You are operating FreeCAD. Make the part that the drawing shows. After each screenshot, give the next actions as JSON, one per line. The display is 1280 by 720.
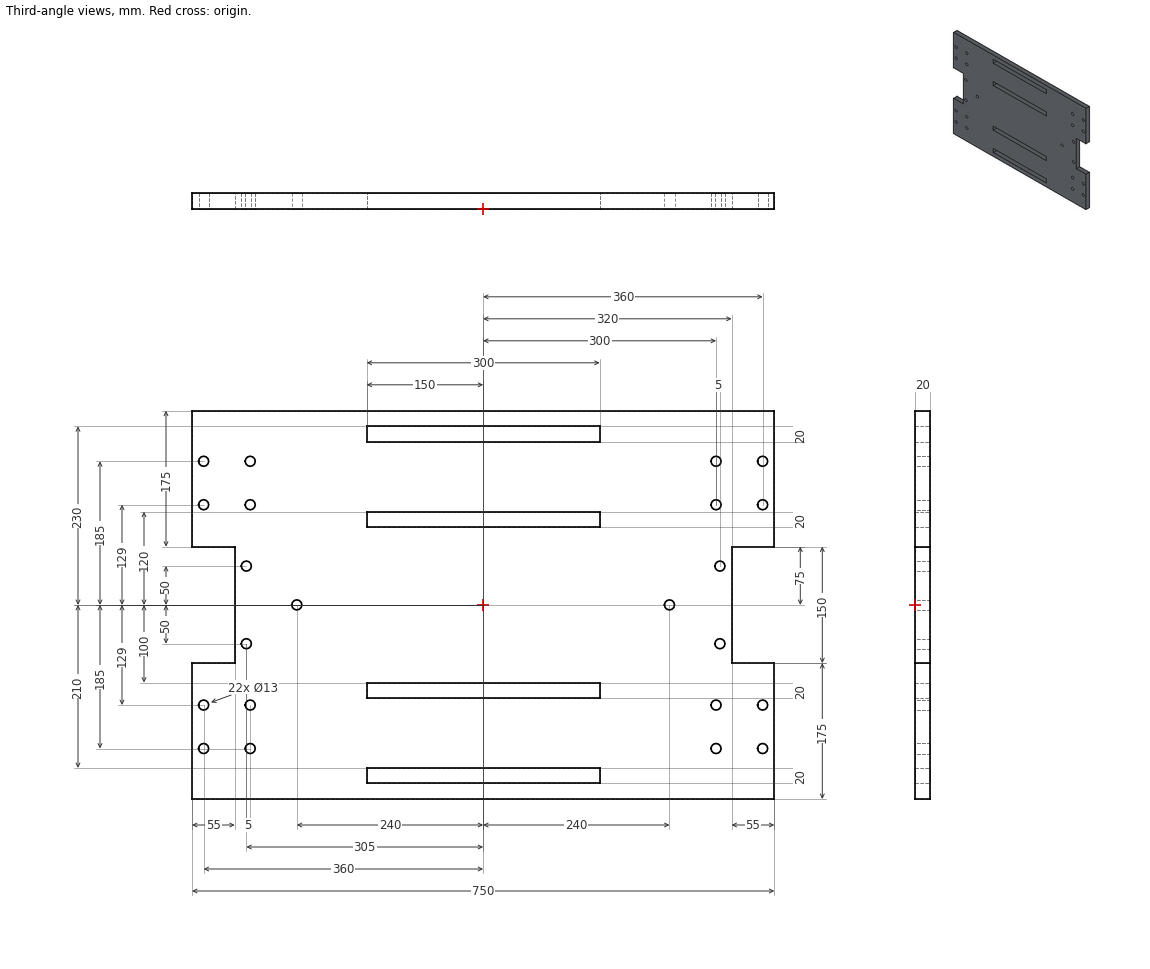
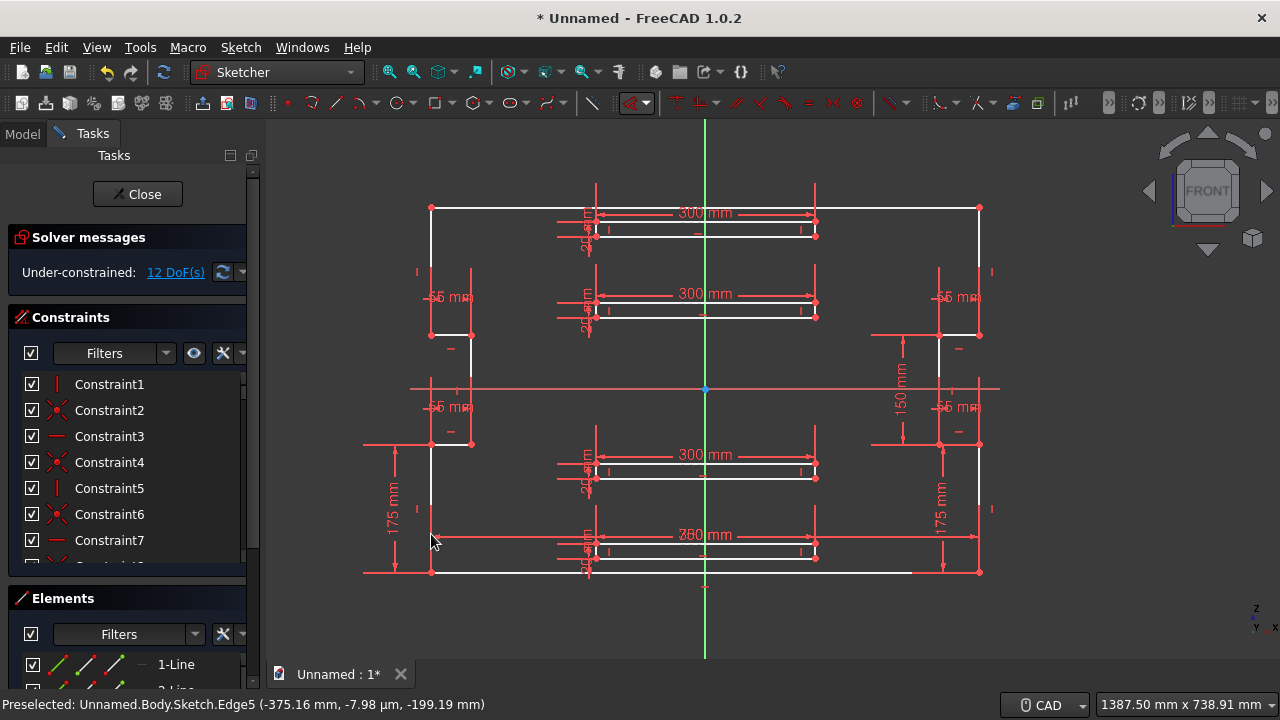
{"action": "left_click", "coordinate": [471, 368]}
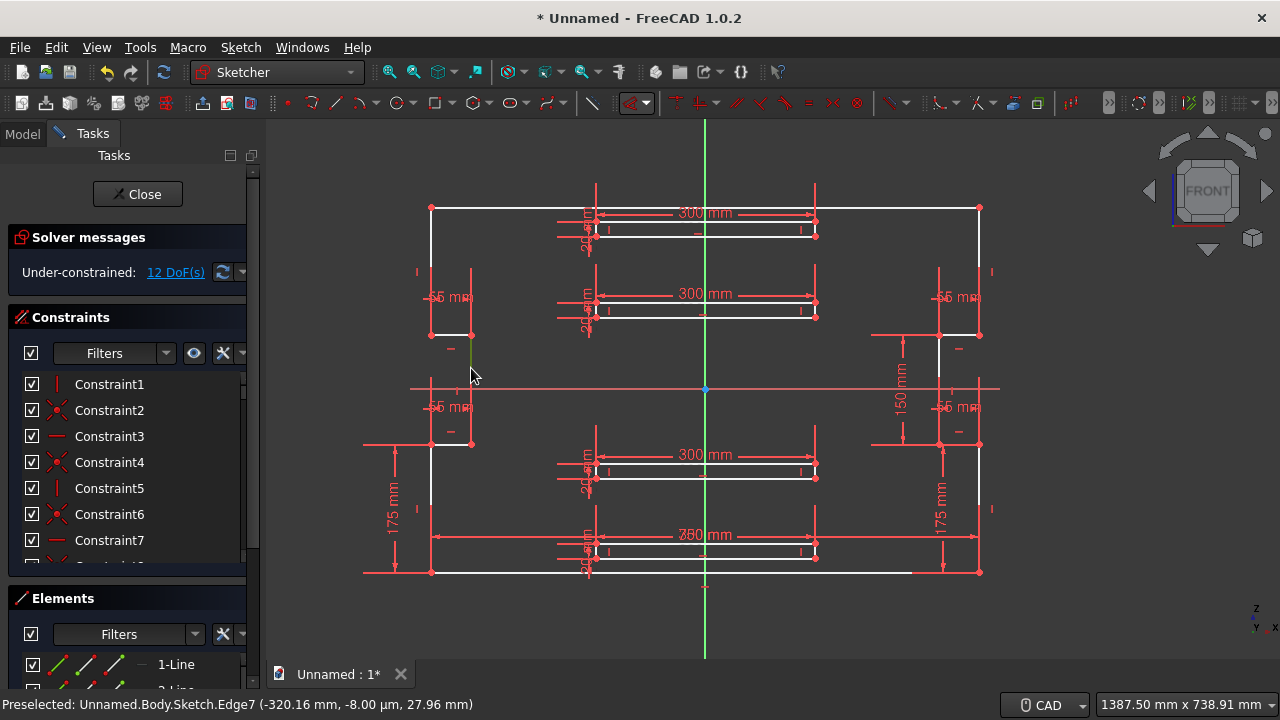
{"action": "left_click", "coordinate": [648, 104]}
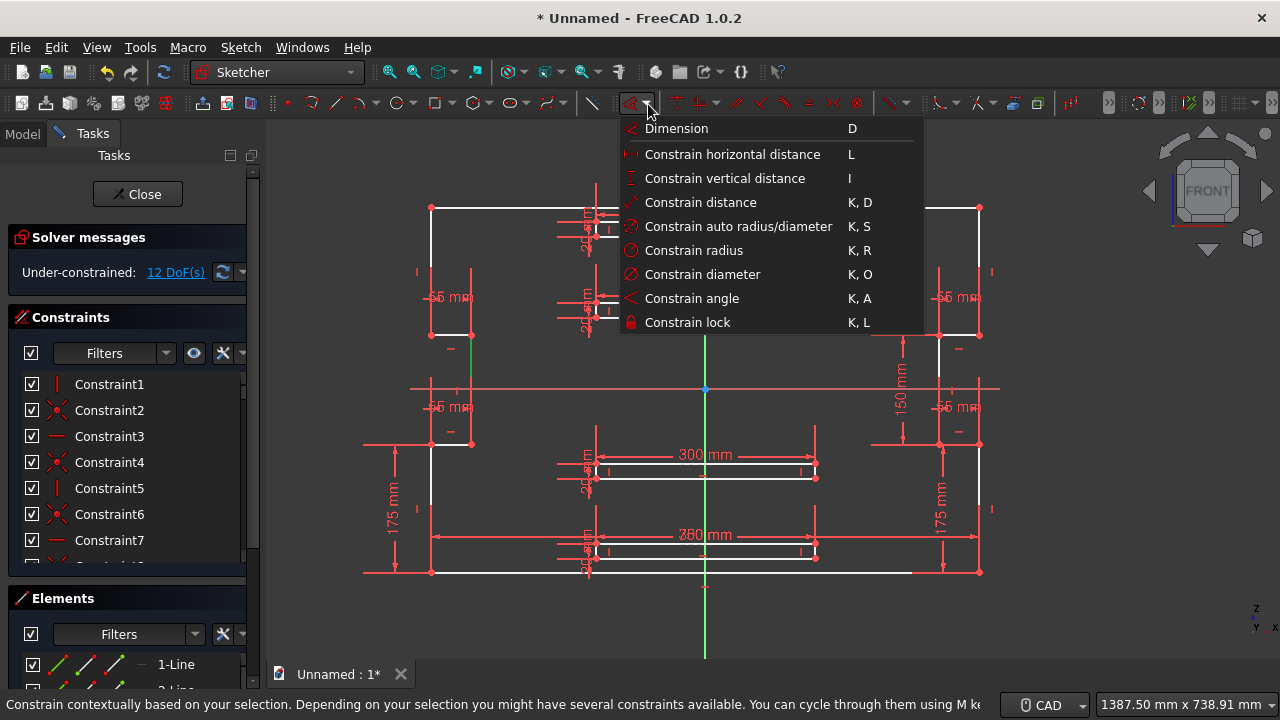
{"action": "left_click", "coordinate": [772, 178]}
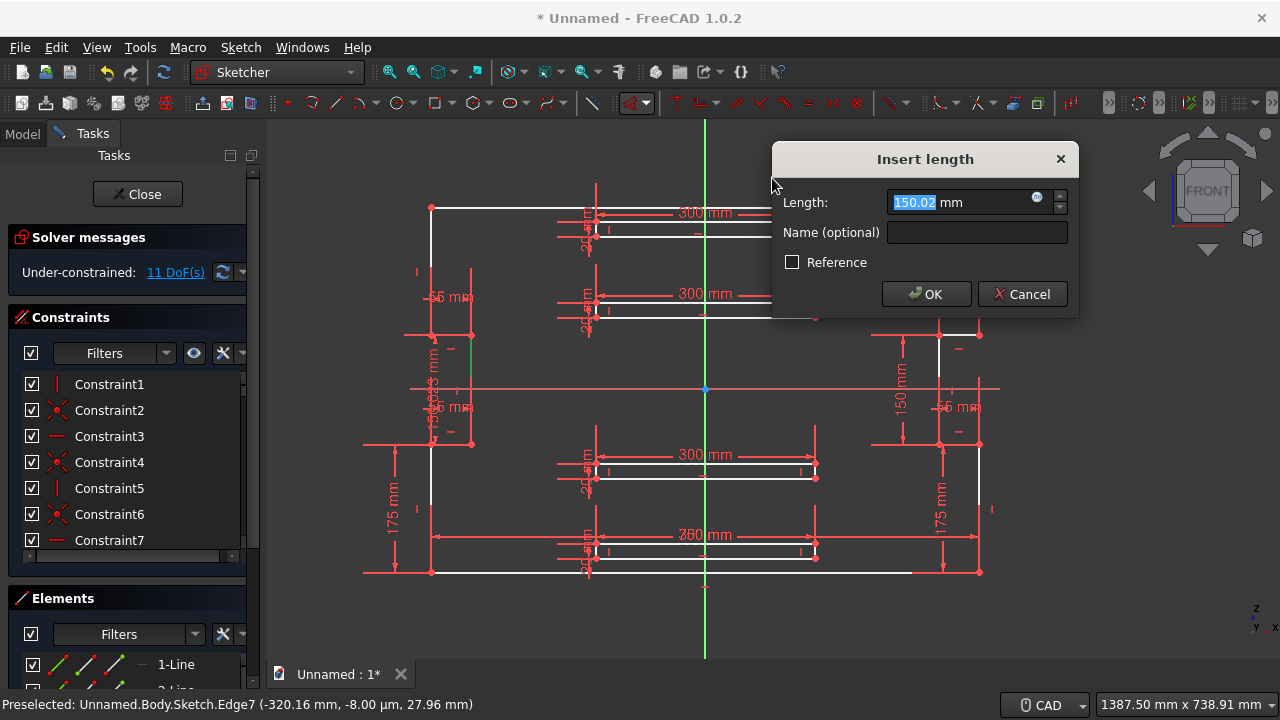
{"action": "type", "text": "150"}
{"action": "key", "text": "Return"}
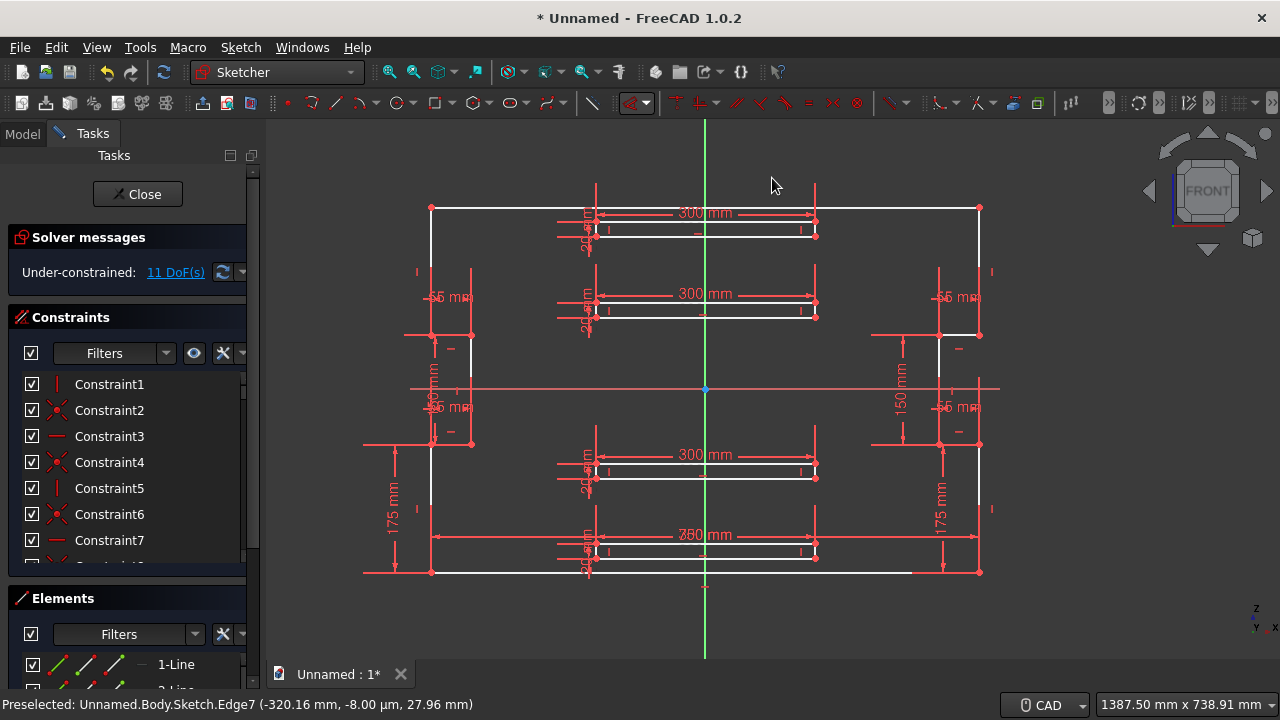
{"action": "left_click", "coordinate": [431, 246]}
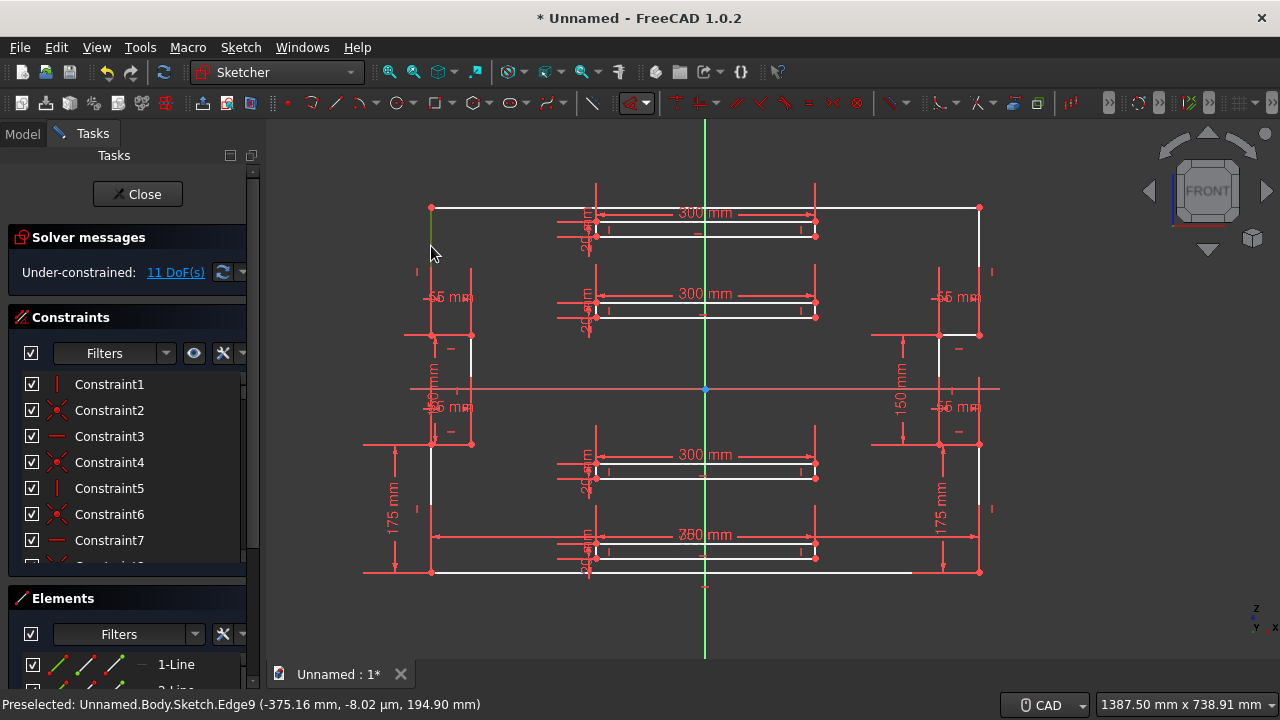
{"action": "key", "text": "i"}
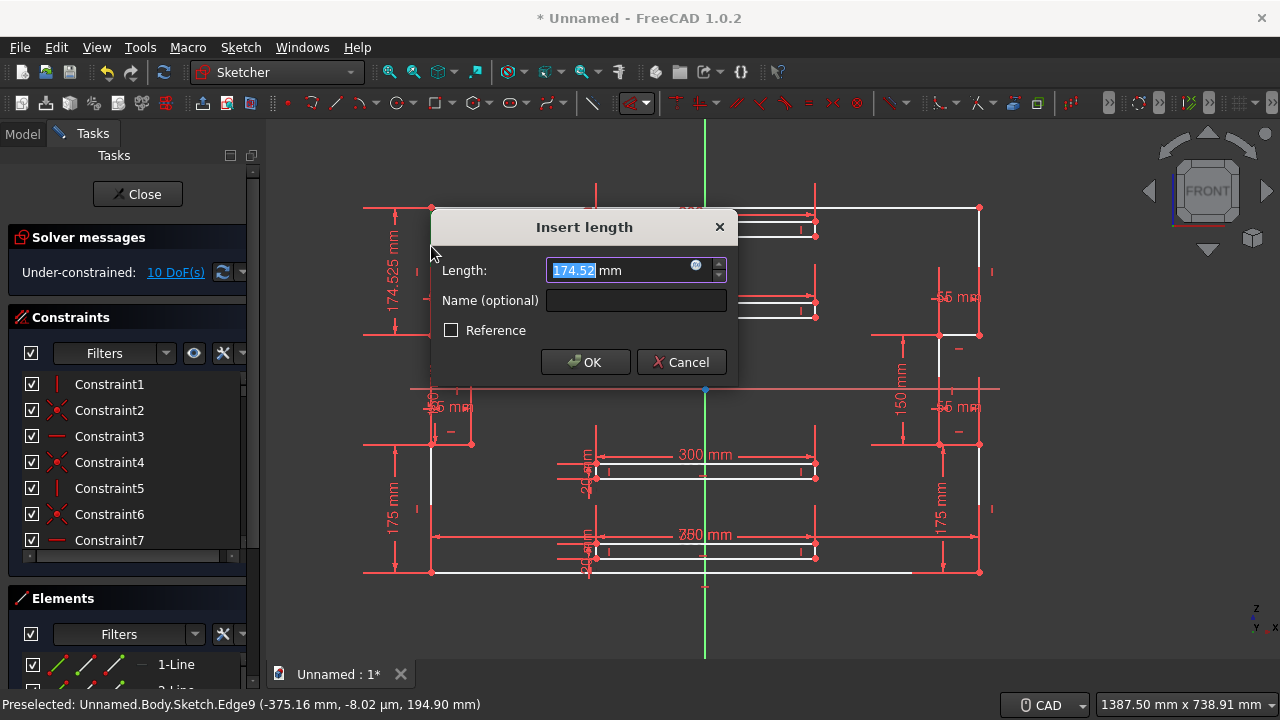
{"action": "type", "text": "175"}
{"action": "key", "text": "Return"}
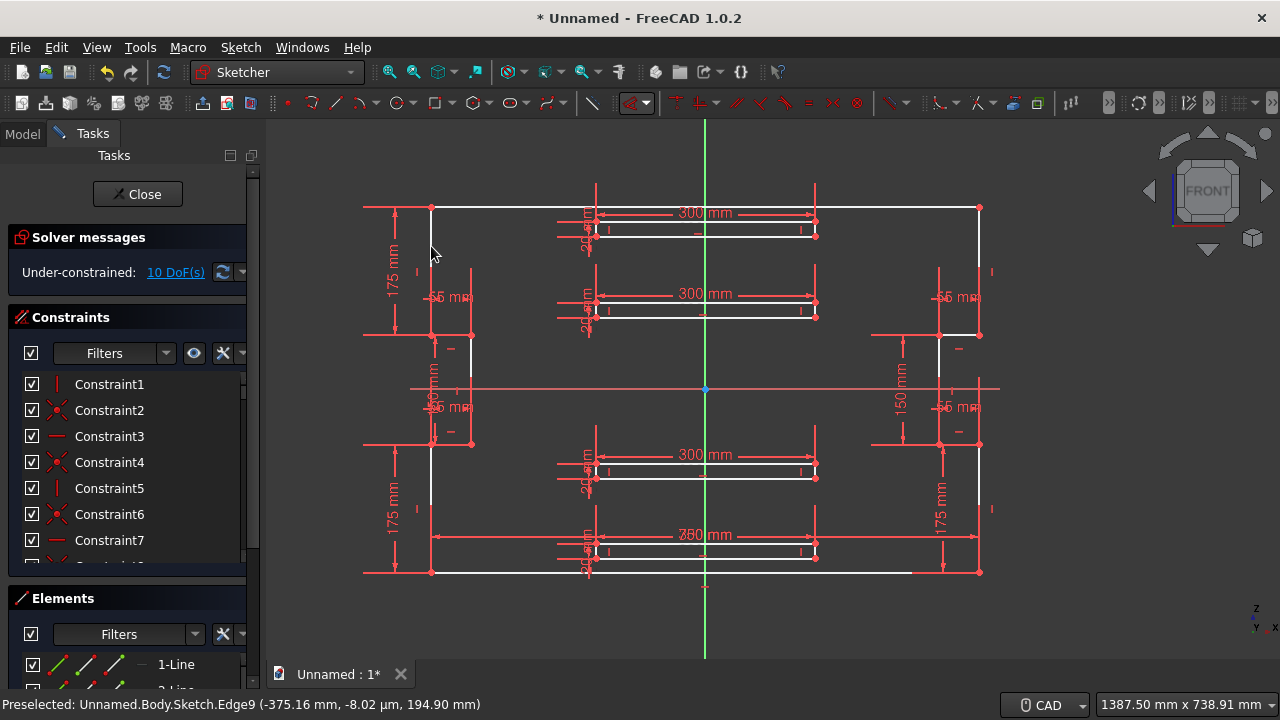
{"action": "left_click", "coordinate": [939, 335]}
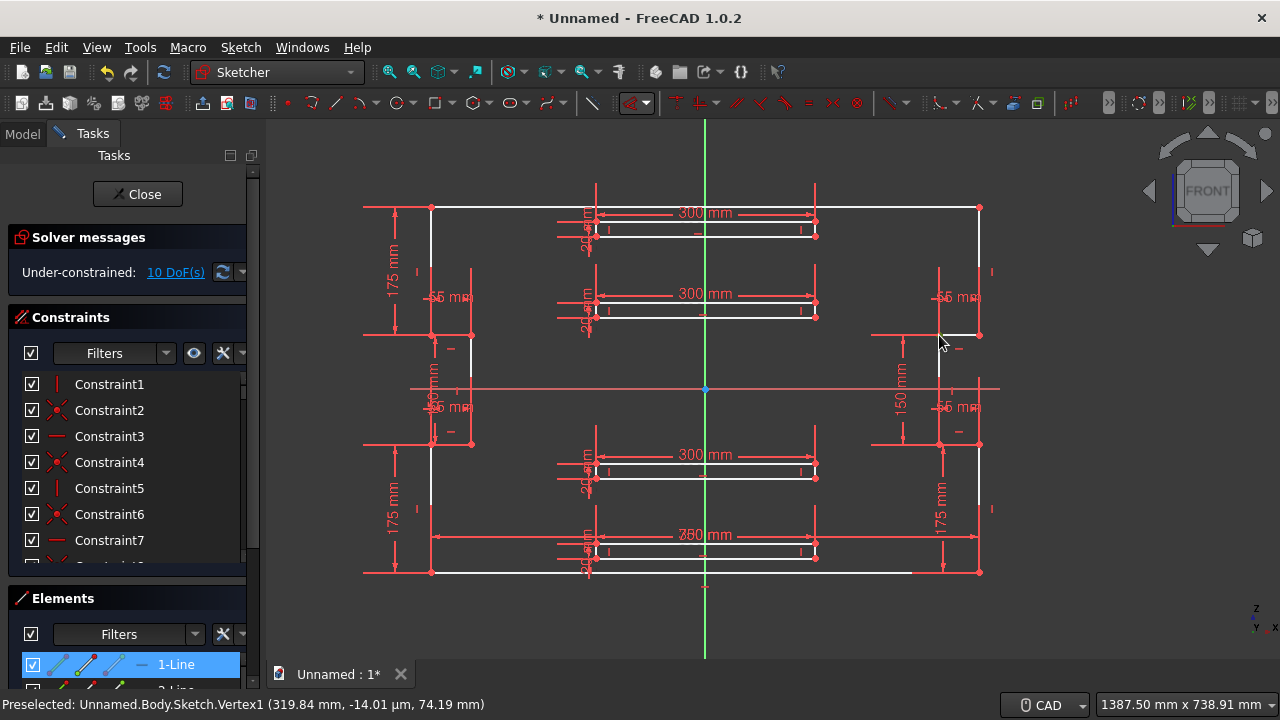
{"action": "key", "text": "i"}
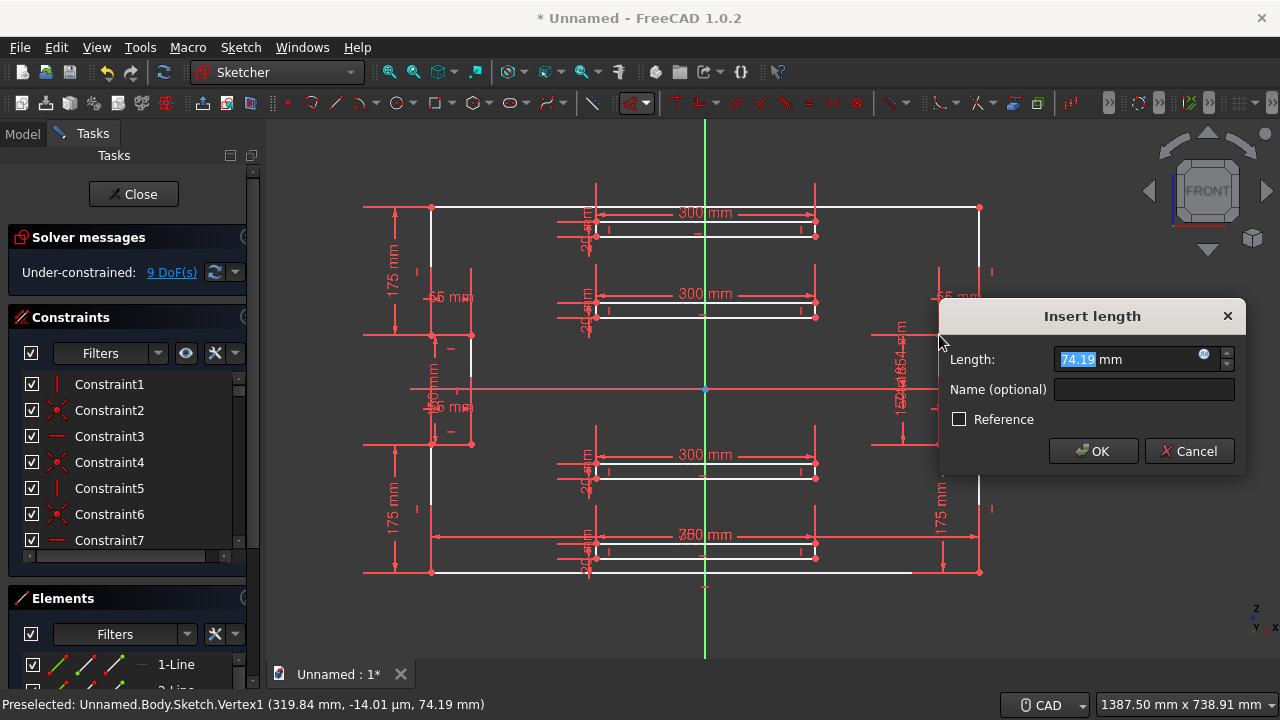
{"action": "type", "text": "75"}
{"action": "key", "text": "Return"}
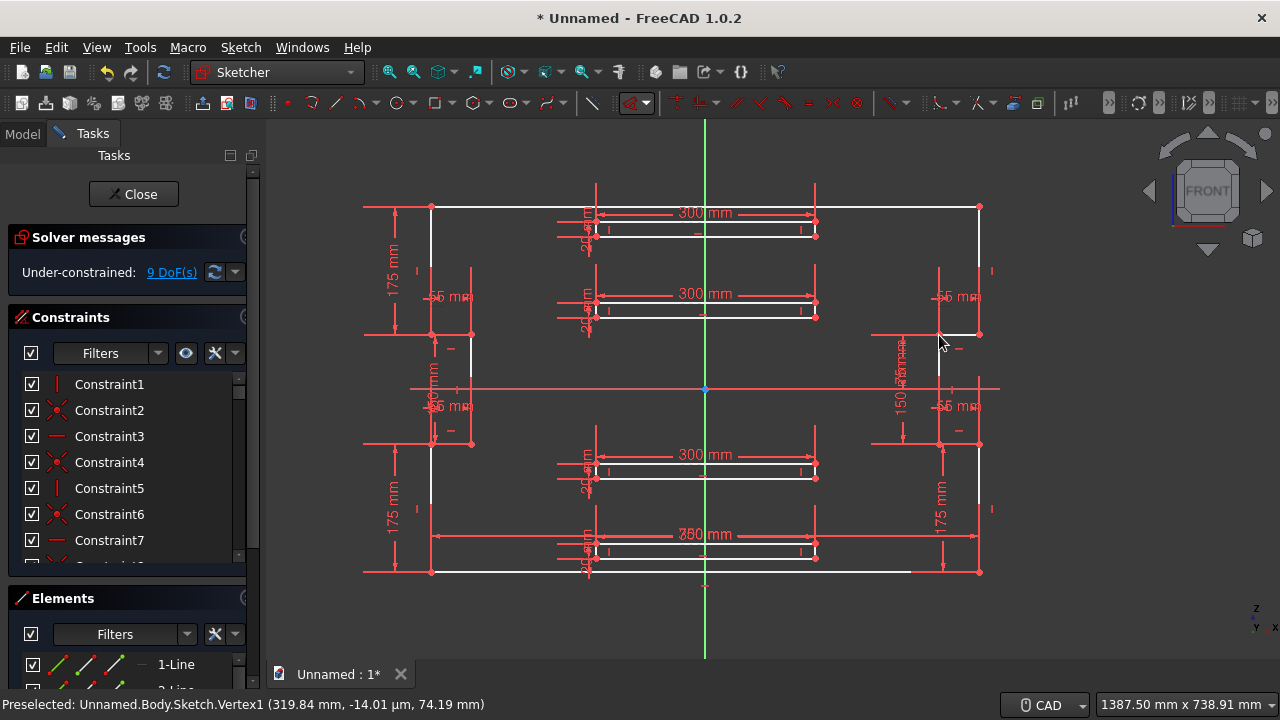
{"action": "left_click", "coordinate": [939, 335]}